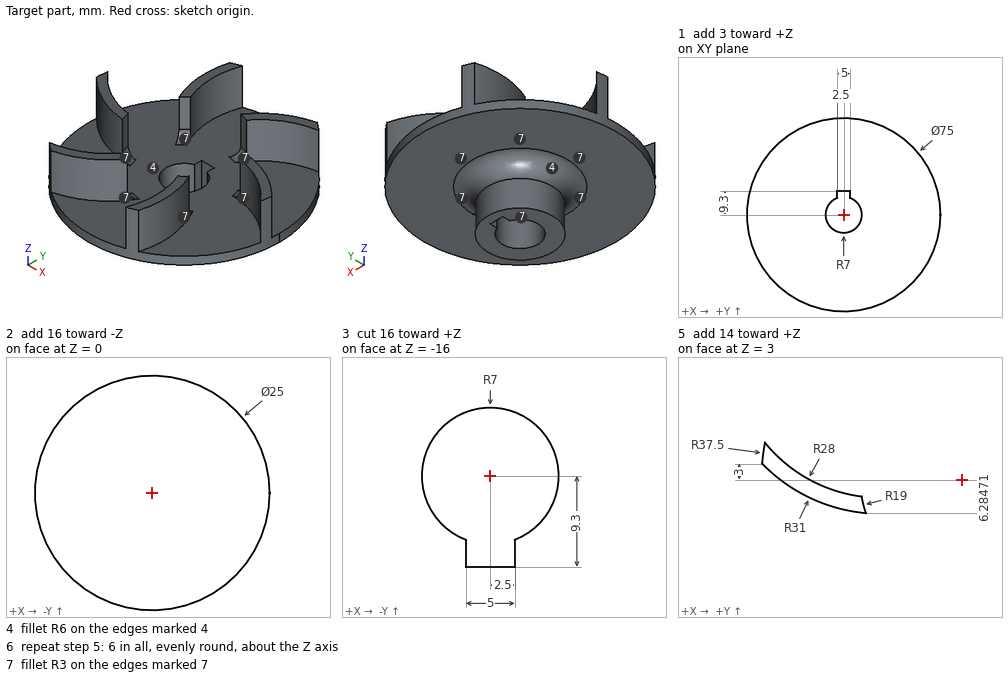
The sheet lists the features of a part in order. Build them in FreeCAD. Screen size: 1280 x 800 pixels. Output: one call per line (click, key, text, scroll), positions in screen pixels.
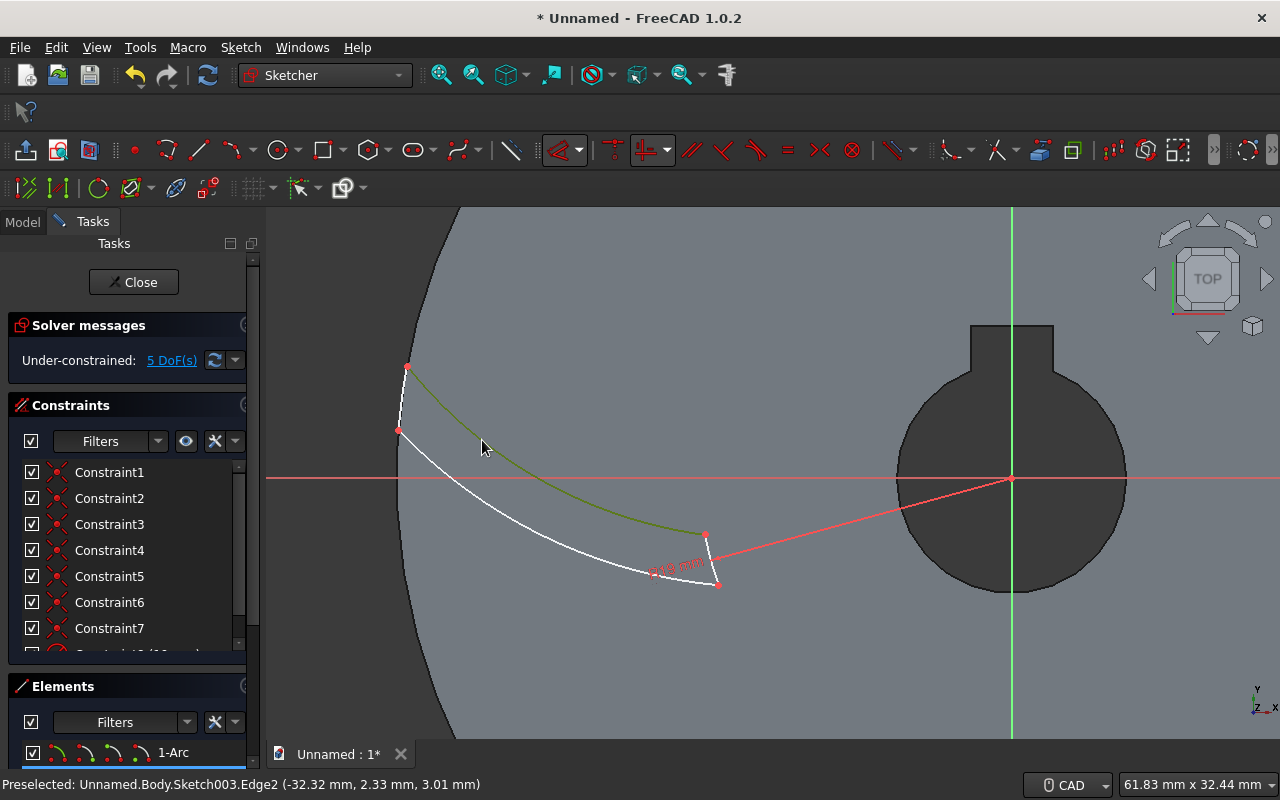
key(k)
key(r)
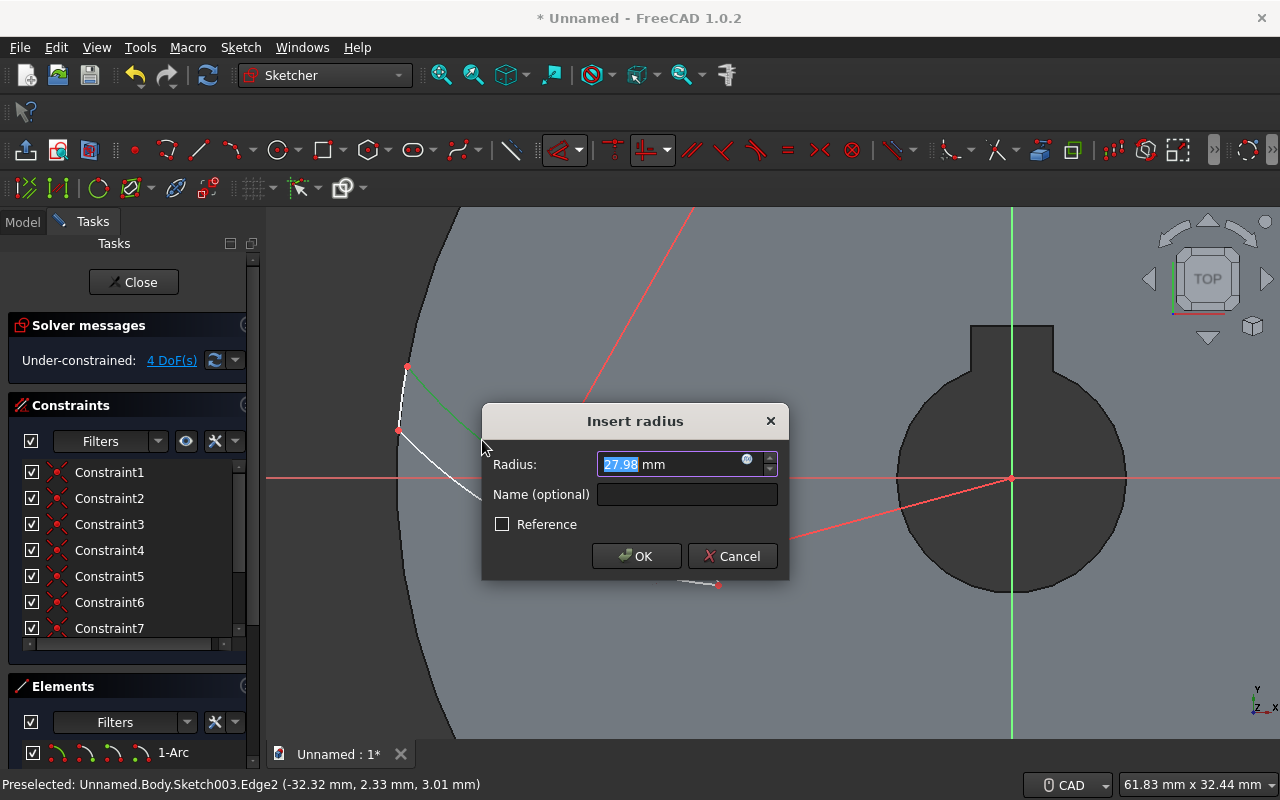
text(28)
key(Return)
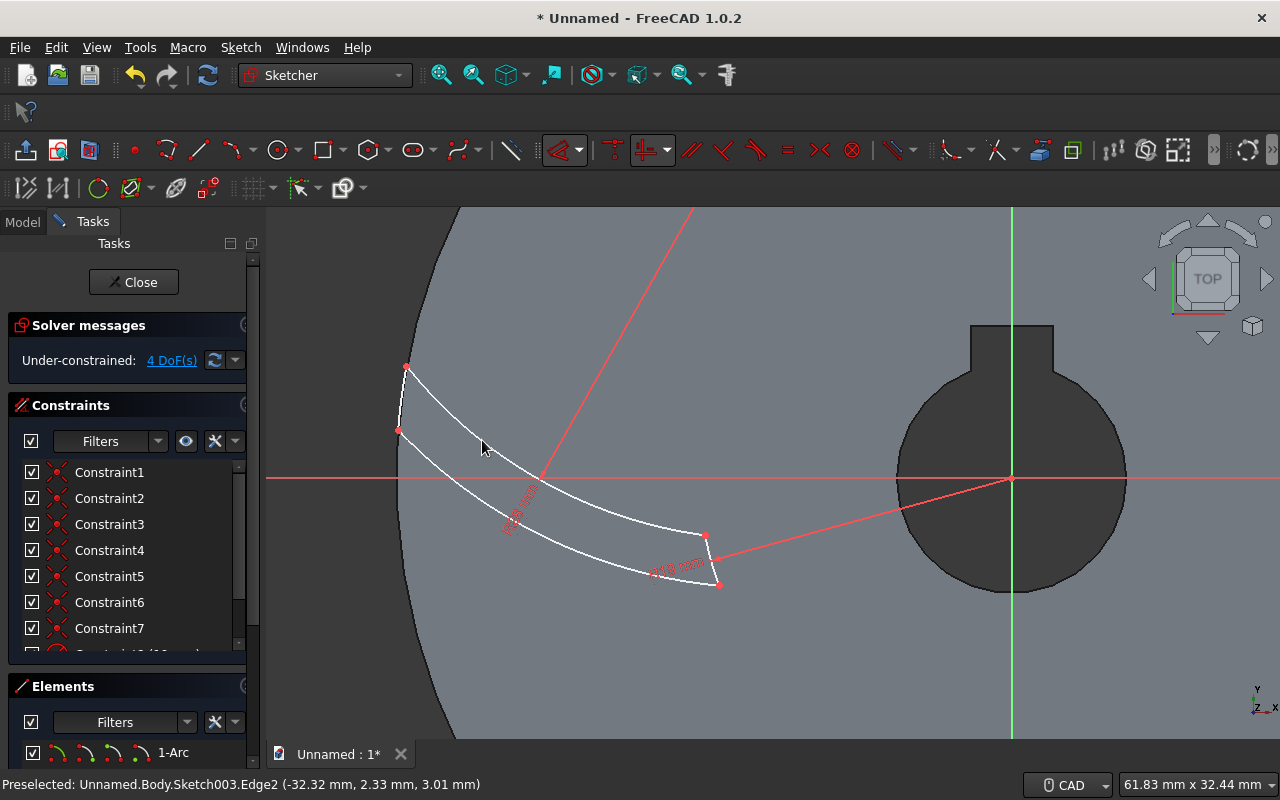
click(403, 385)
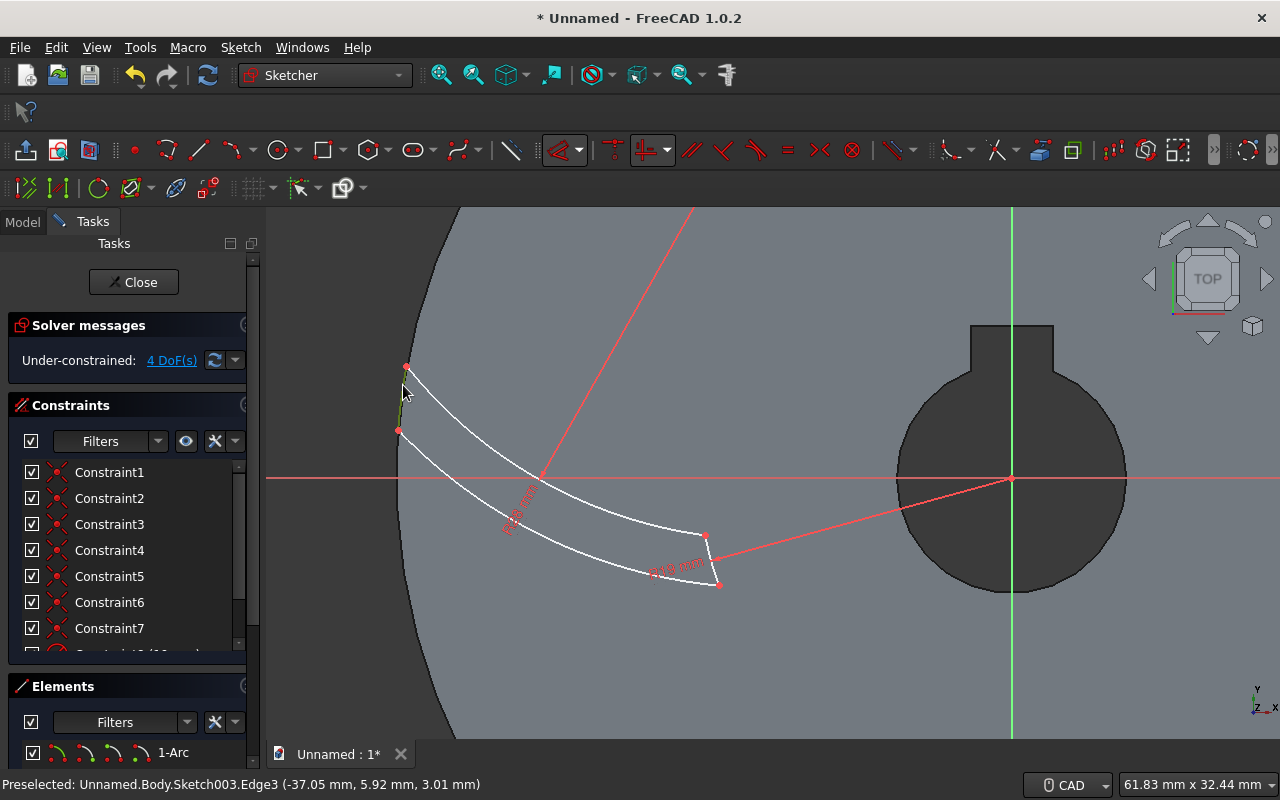
key(k)
key(r)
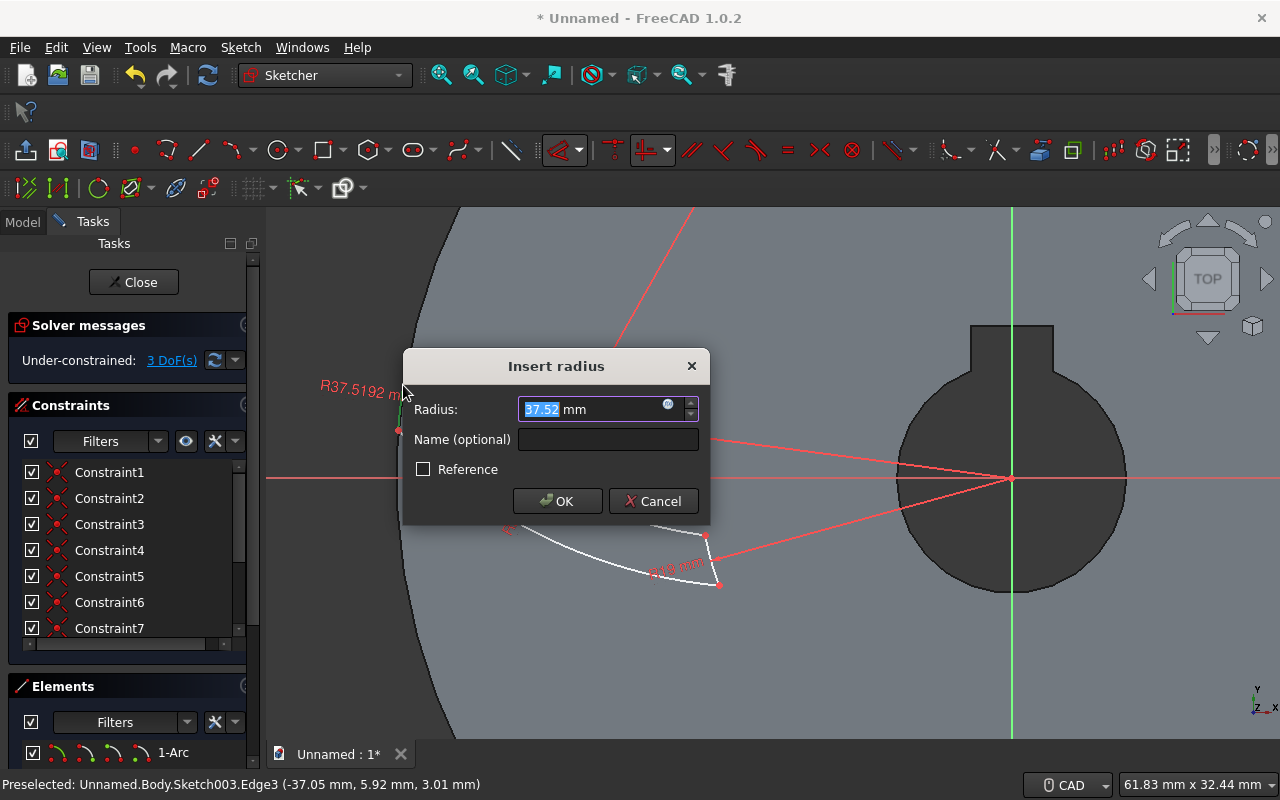
text(37.5)
key(Return)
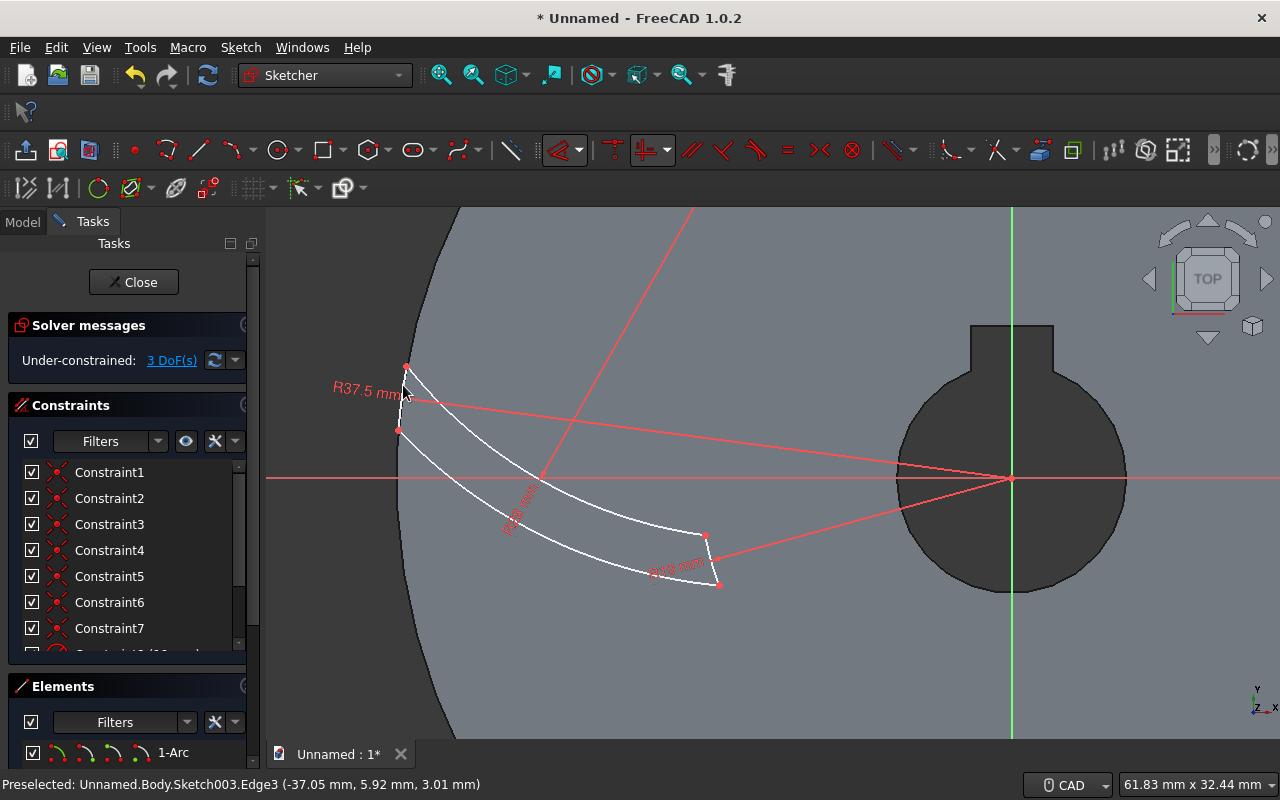
click(482, 500)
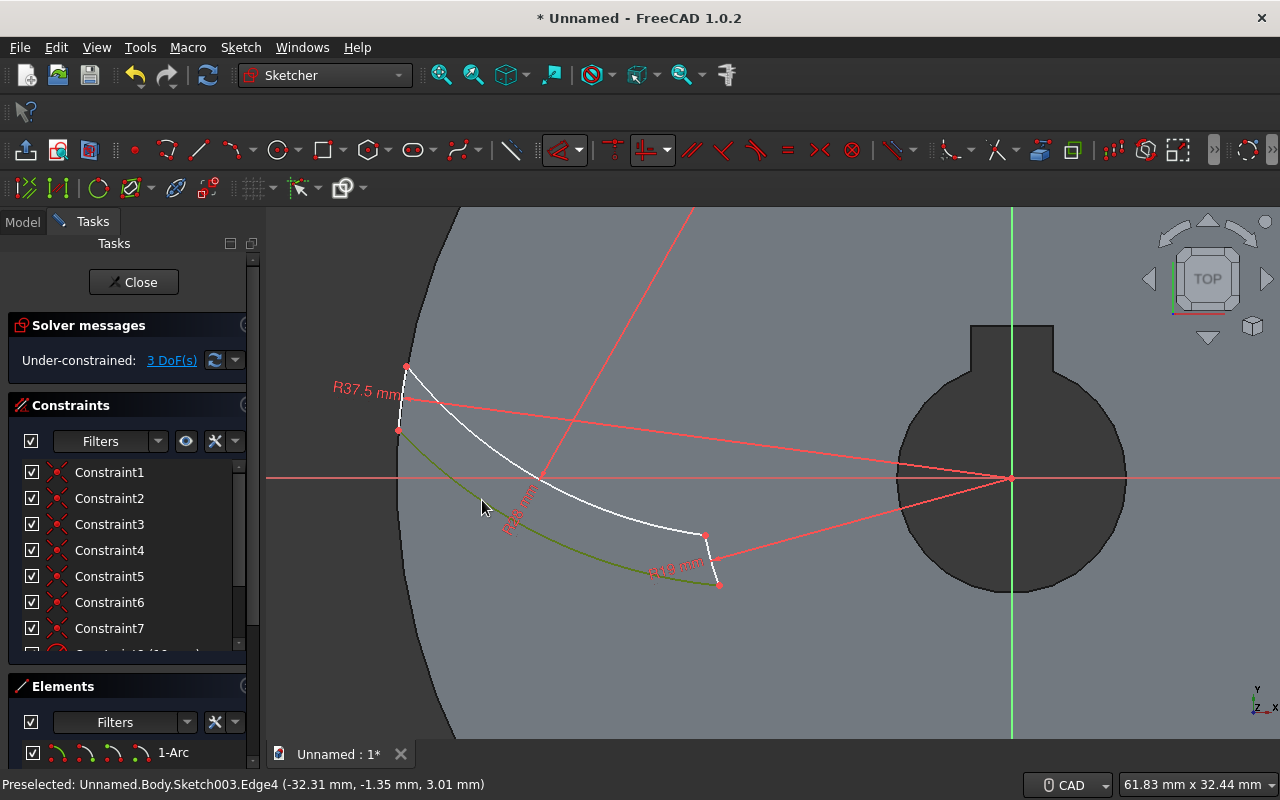
key(k)
key(r)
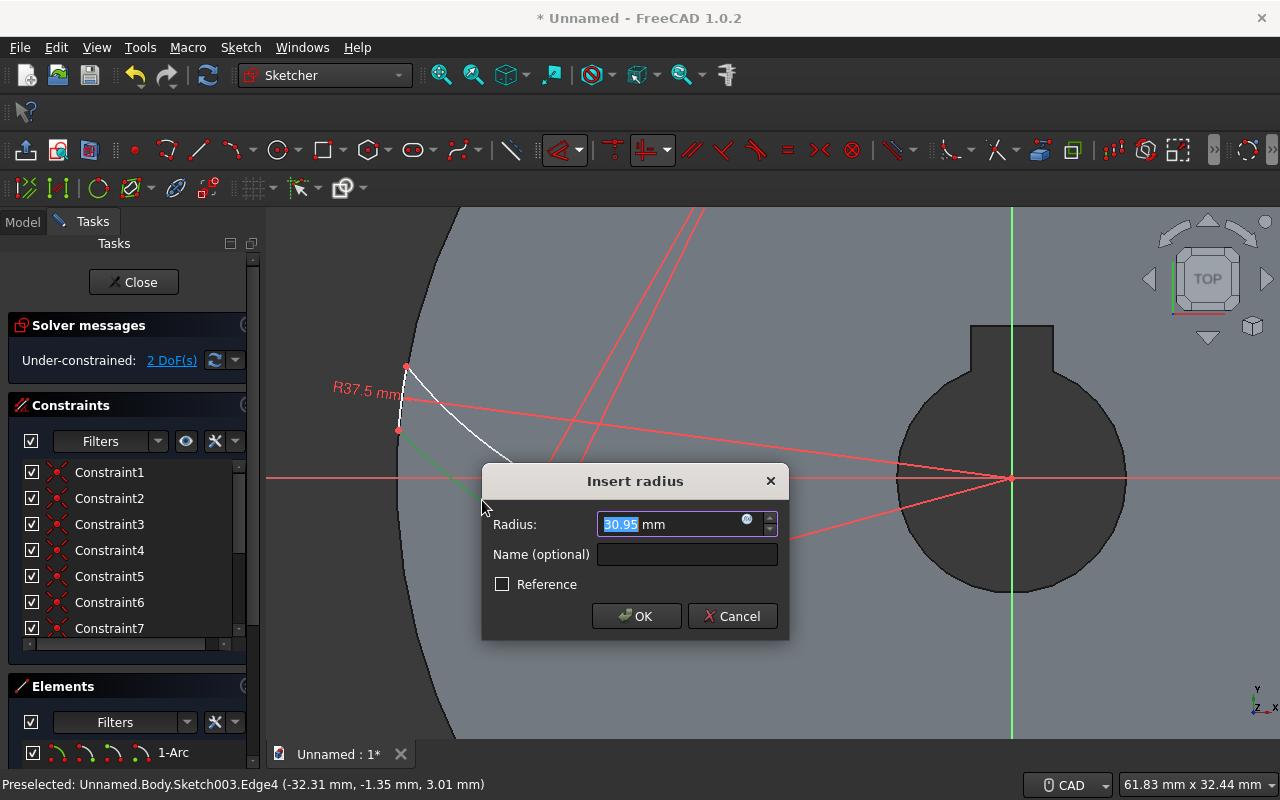
text(31)
key(Return)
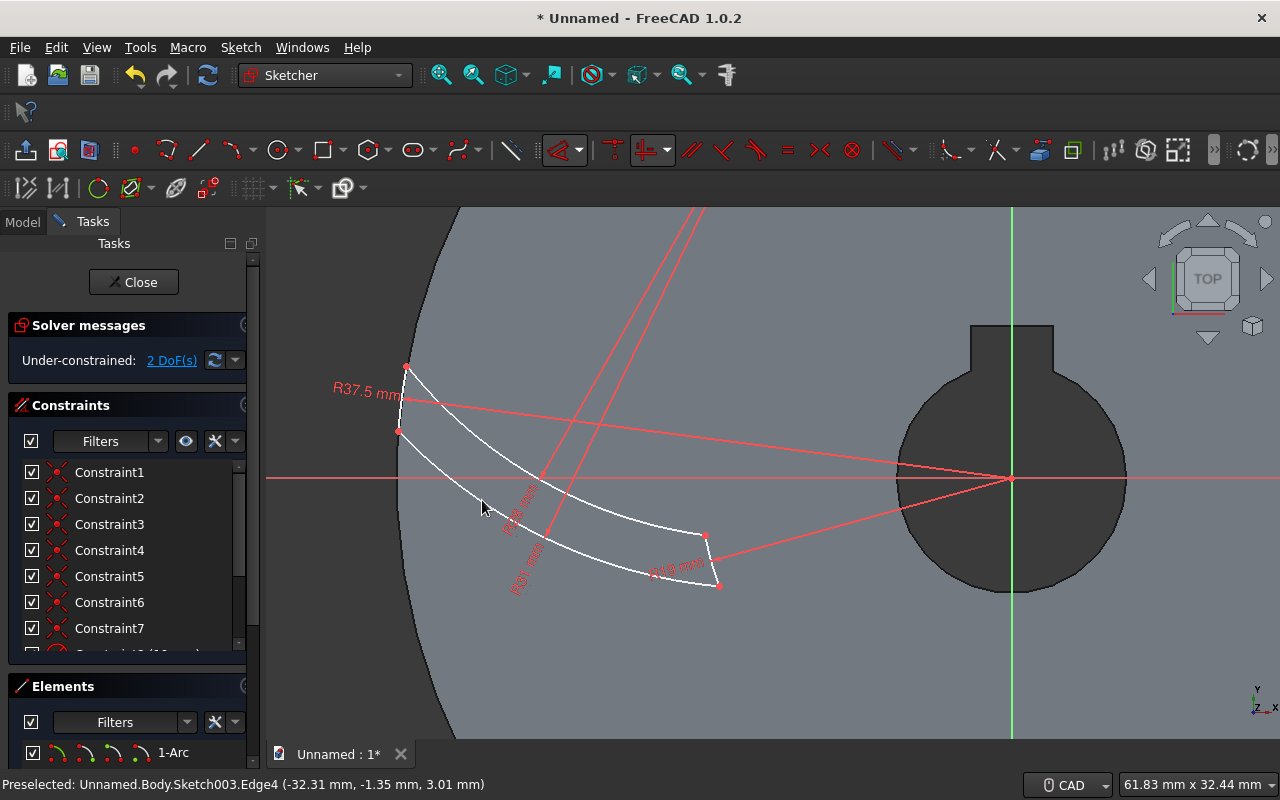
click(398, 431)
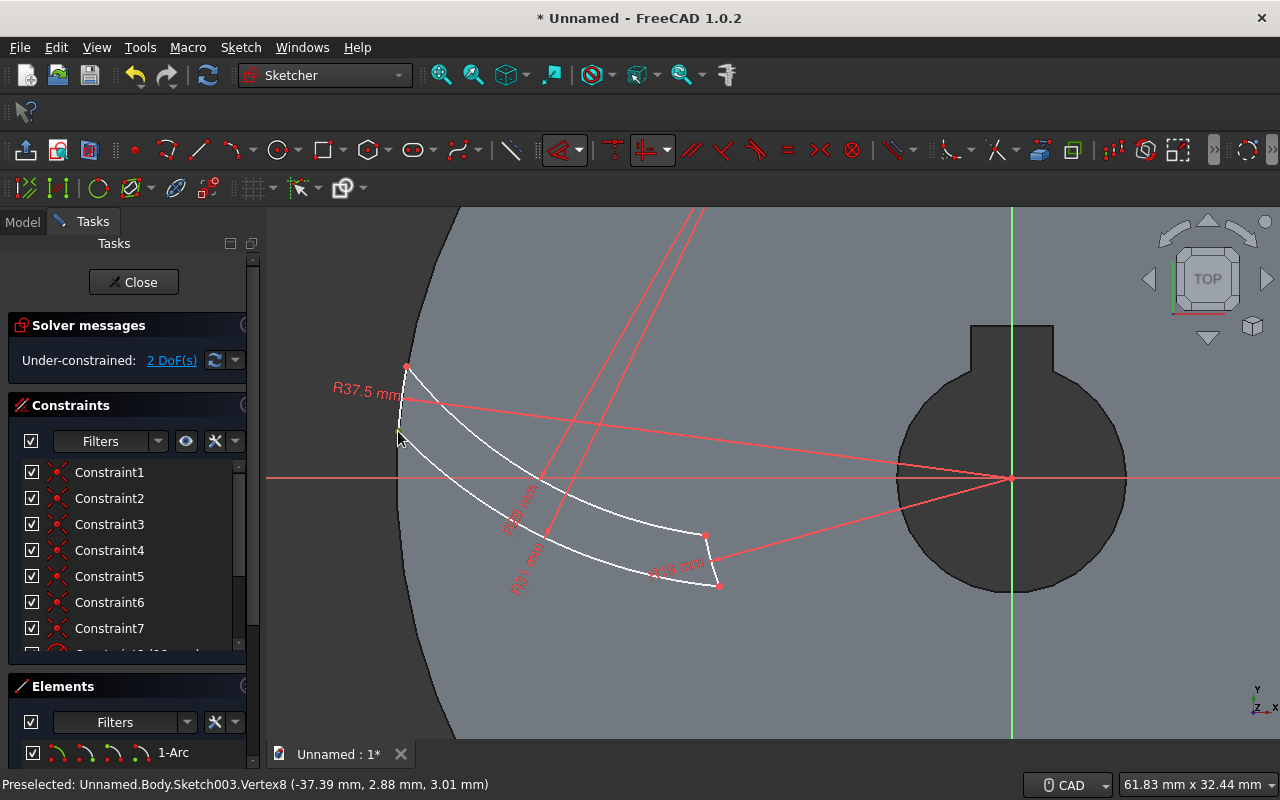
key(i)